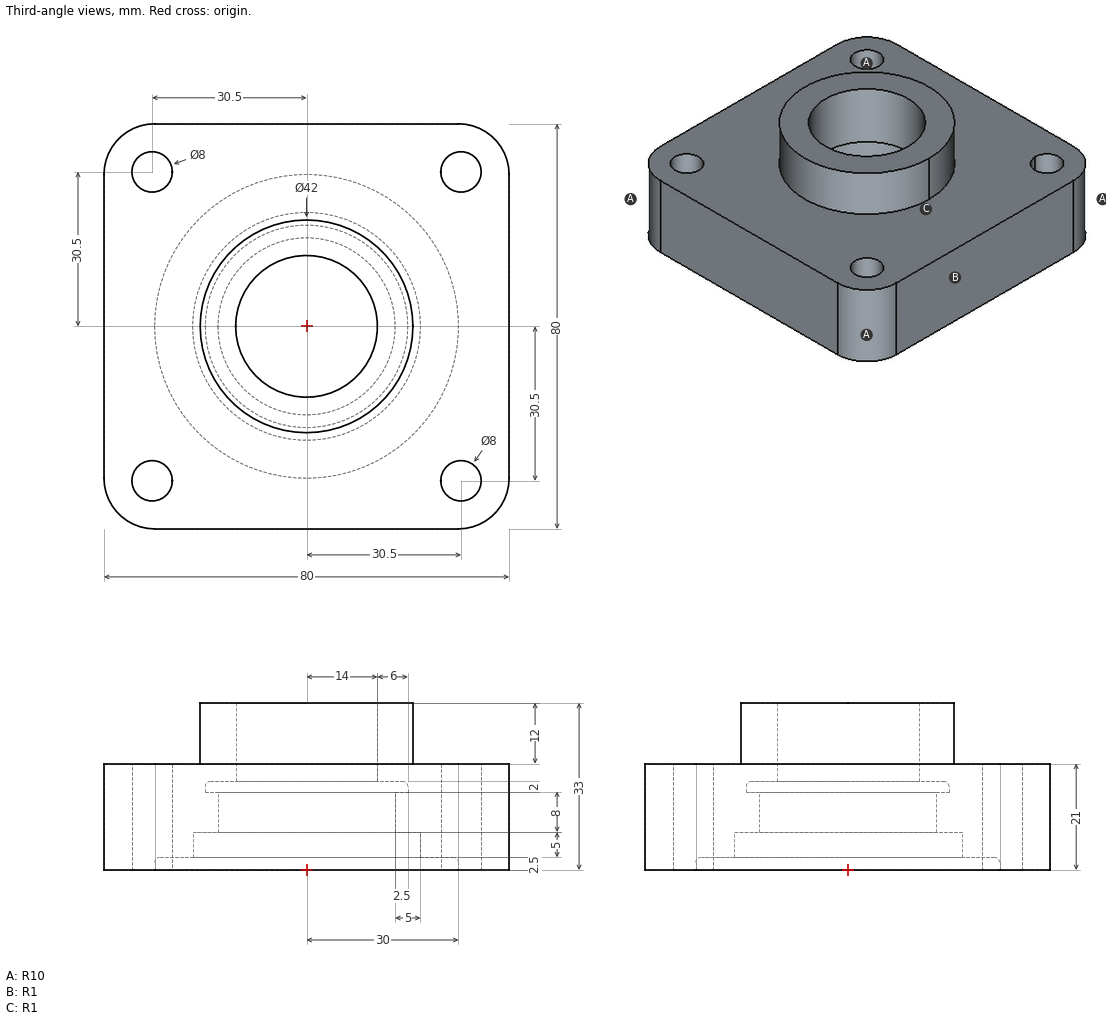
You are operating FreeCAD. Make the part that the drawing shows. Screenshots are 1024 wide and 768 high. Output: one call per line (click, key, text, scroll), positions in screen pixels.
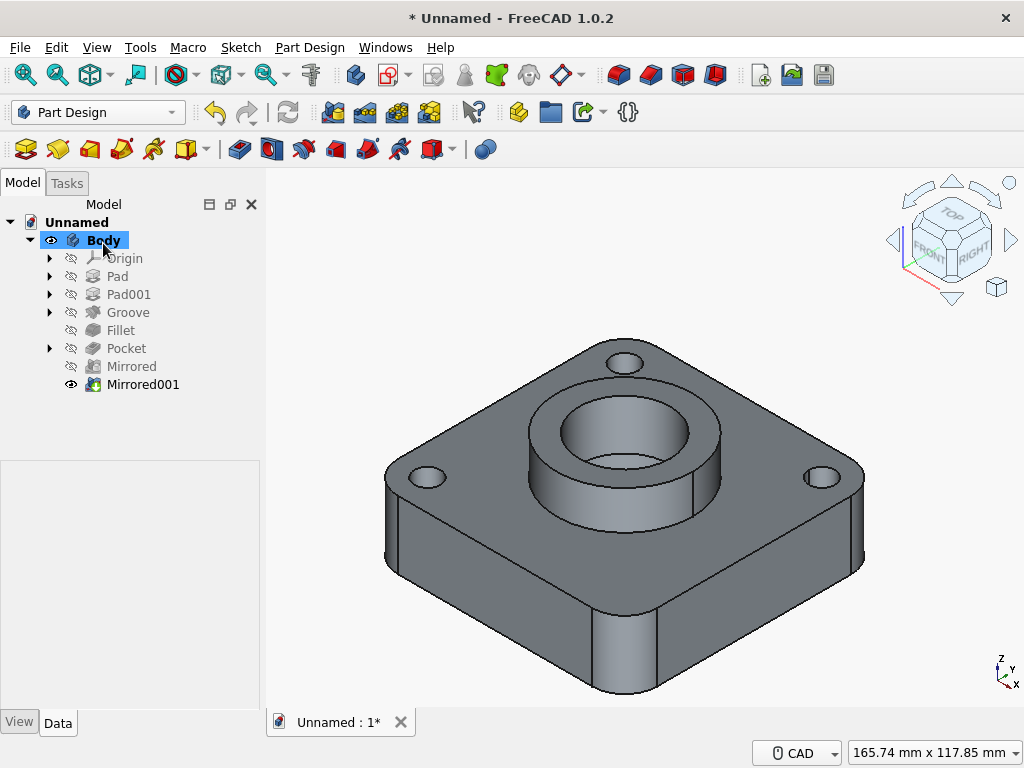
click(625, 562)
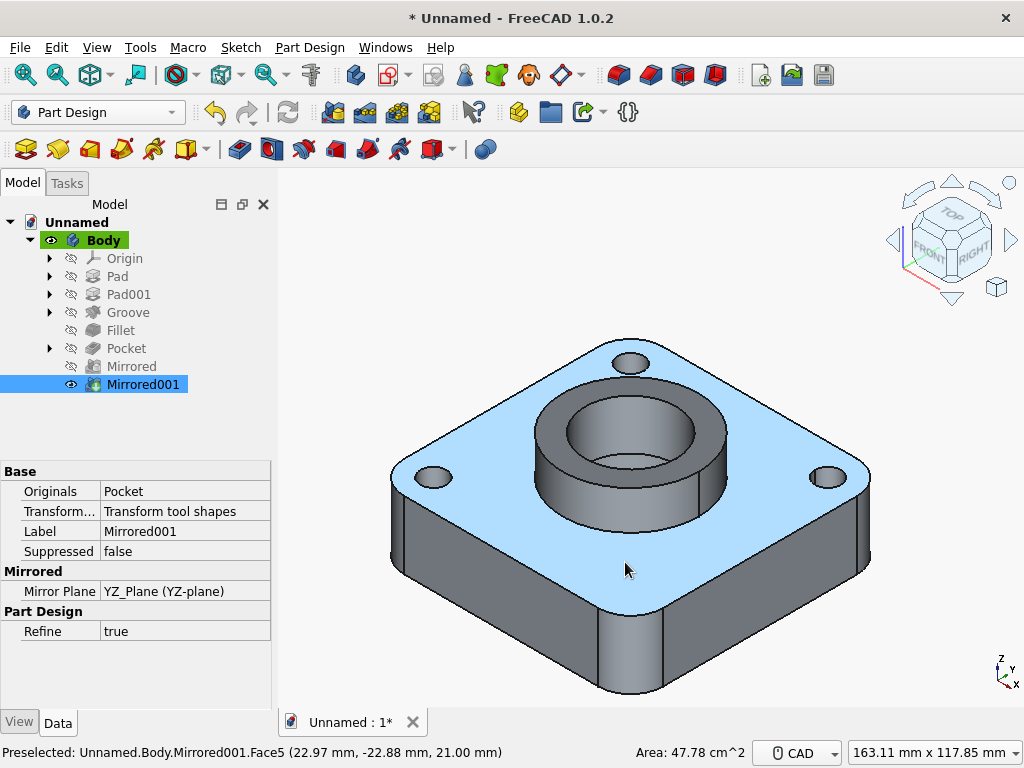
click(388, 76)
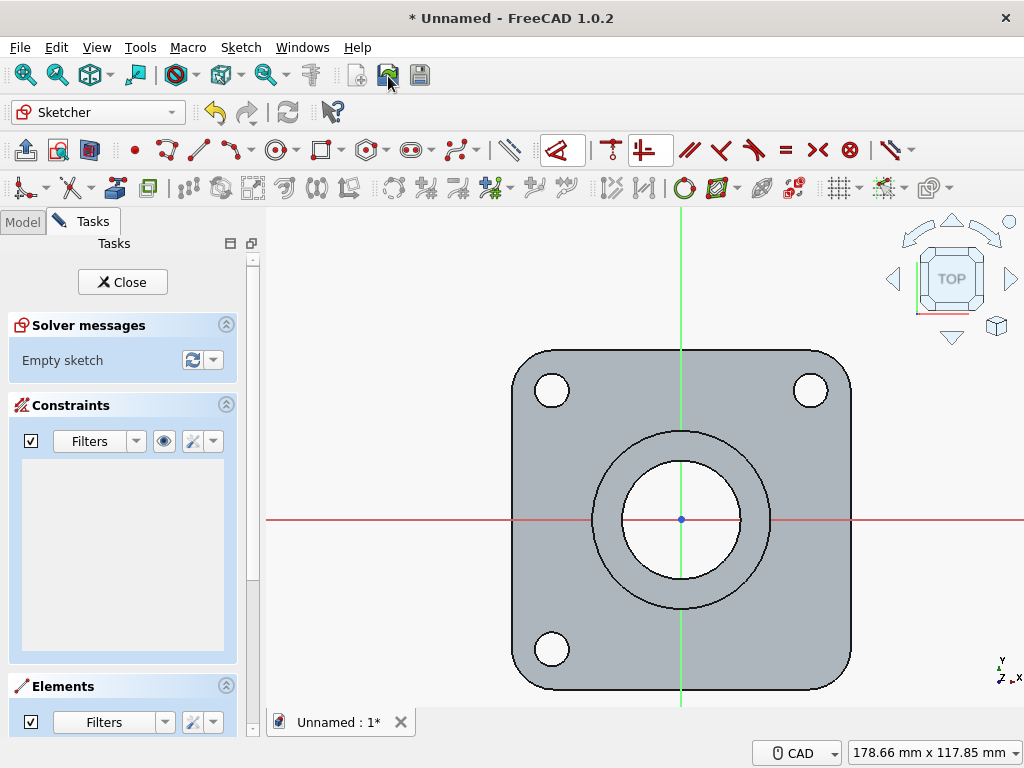
click(90, 150)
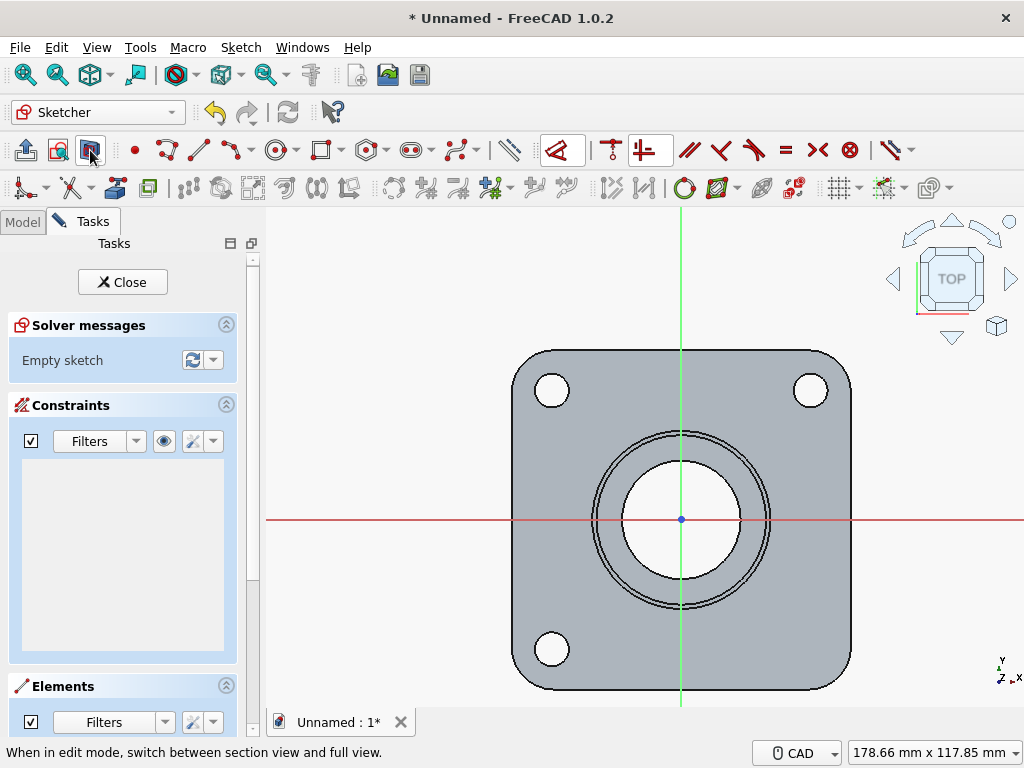
scroll(840, 673, up, 11)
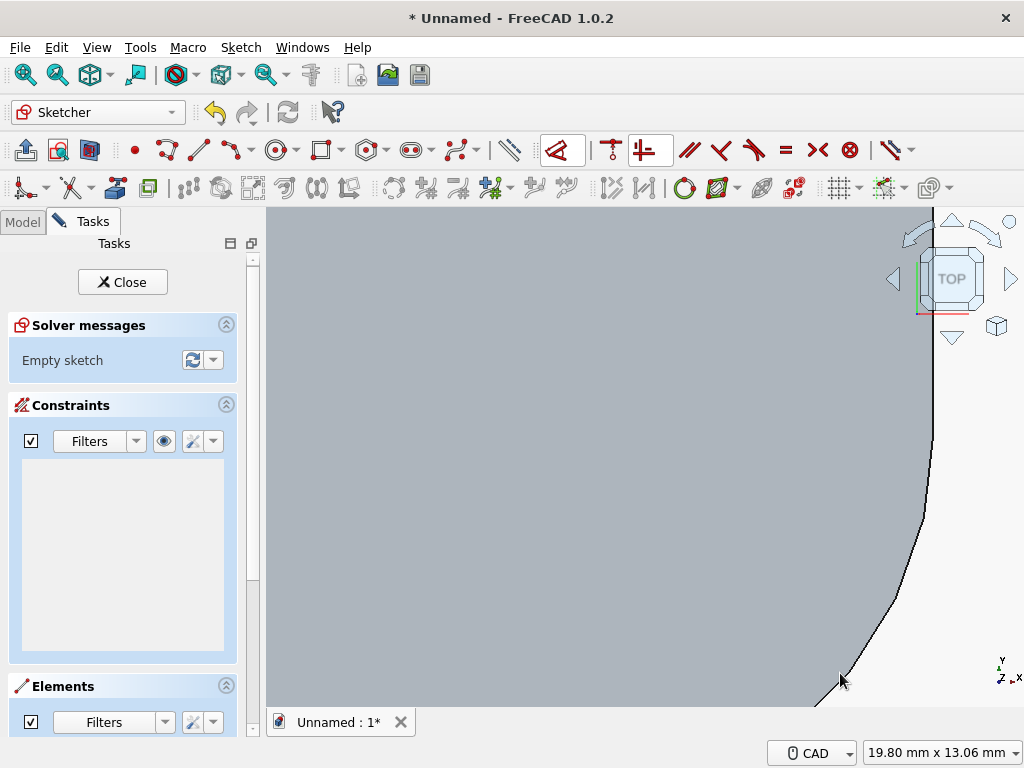
click(276, 150)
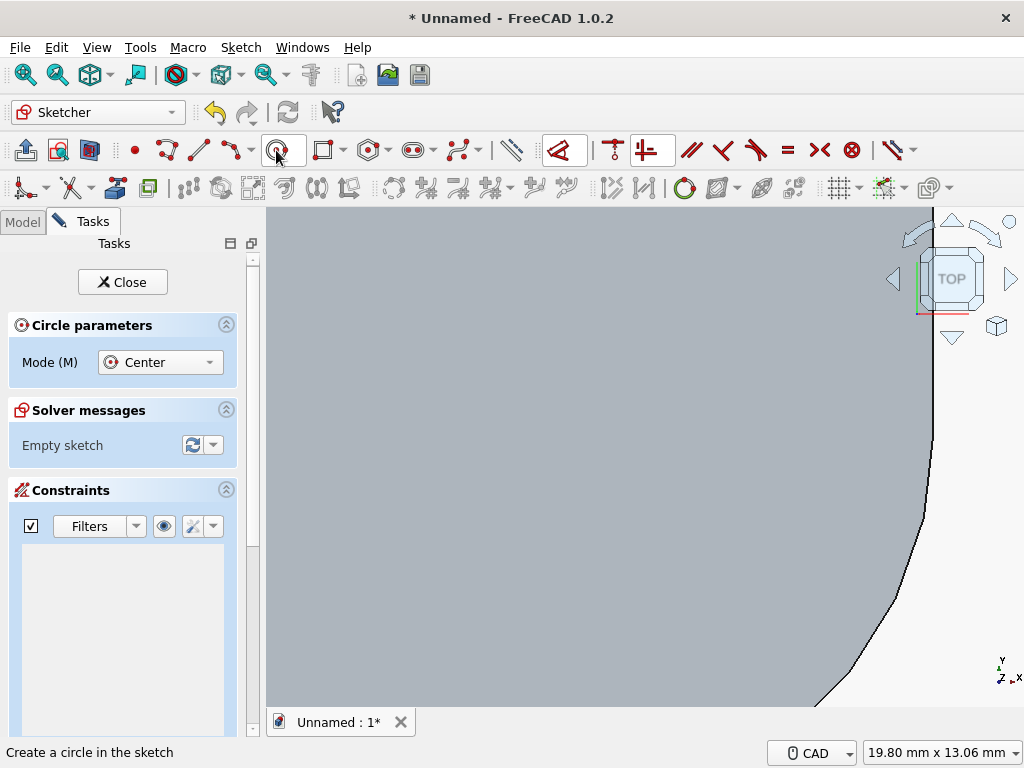
click(570, 452)
move(678, 343)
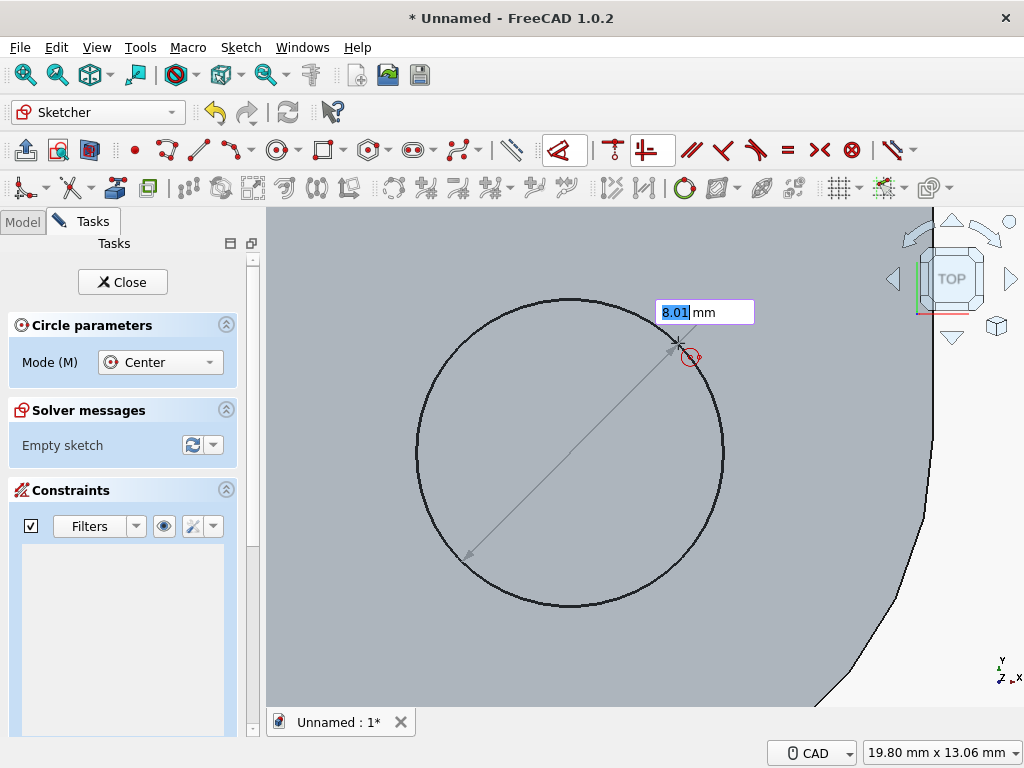
text(8)
key(Return)
key(Escape)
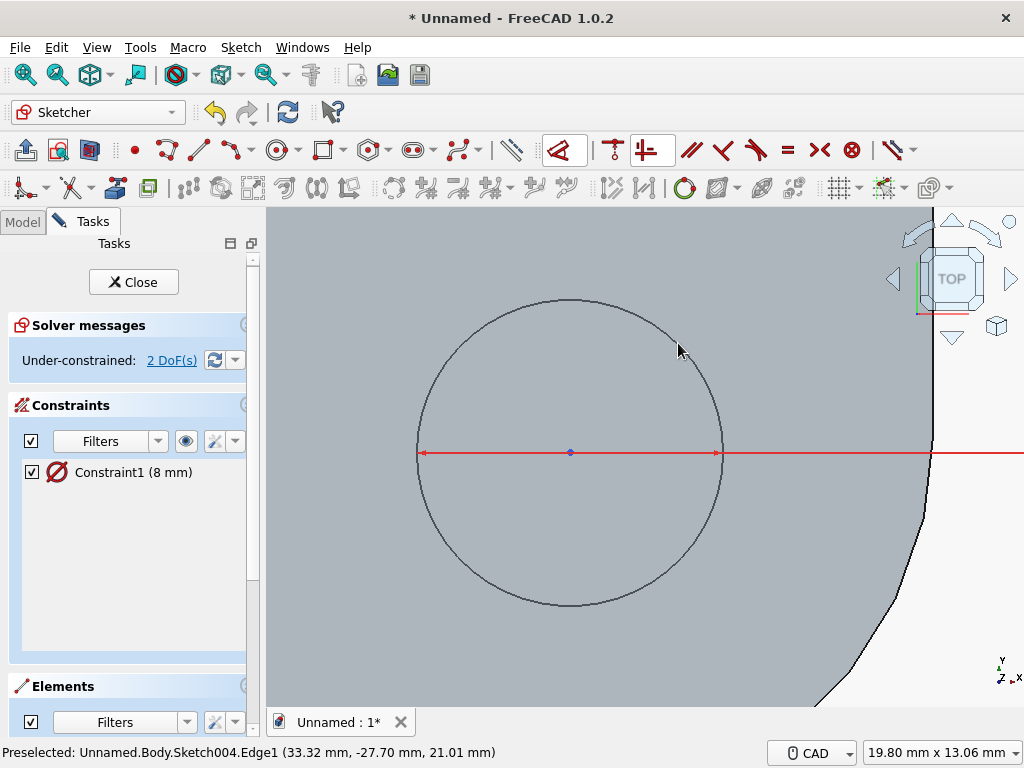
click(570, 453)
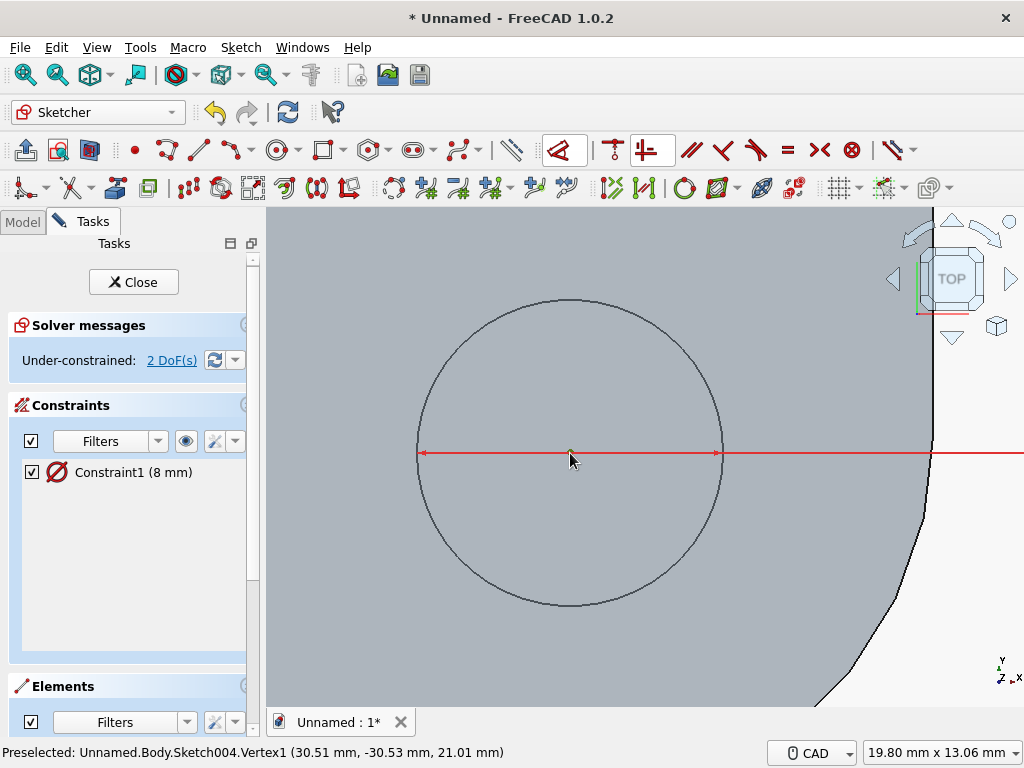
key(l)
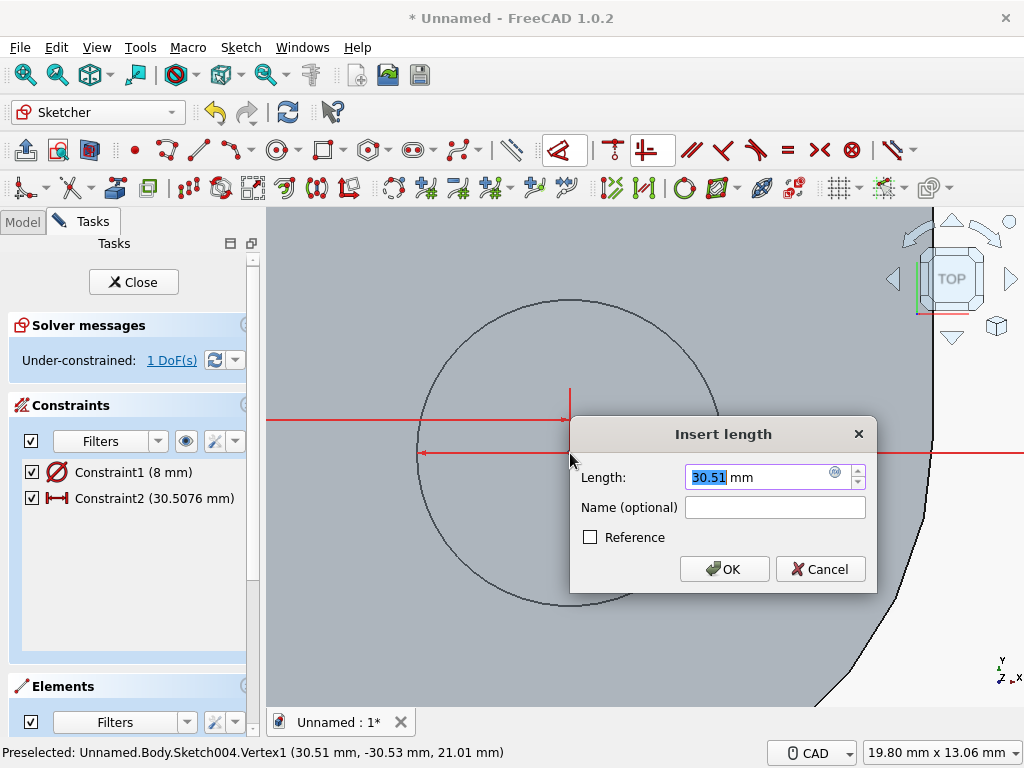
text(30.5)
key(Return)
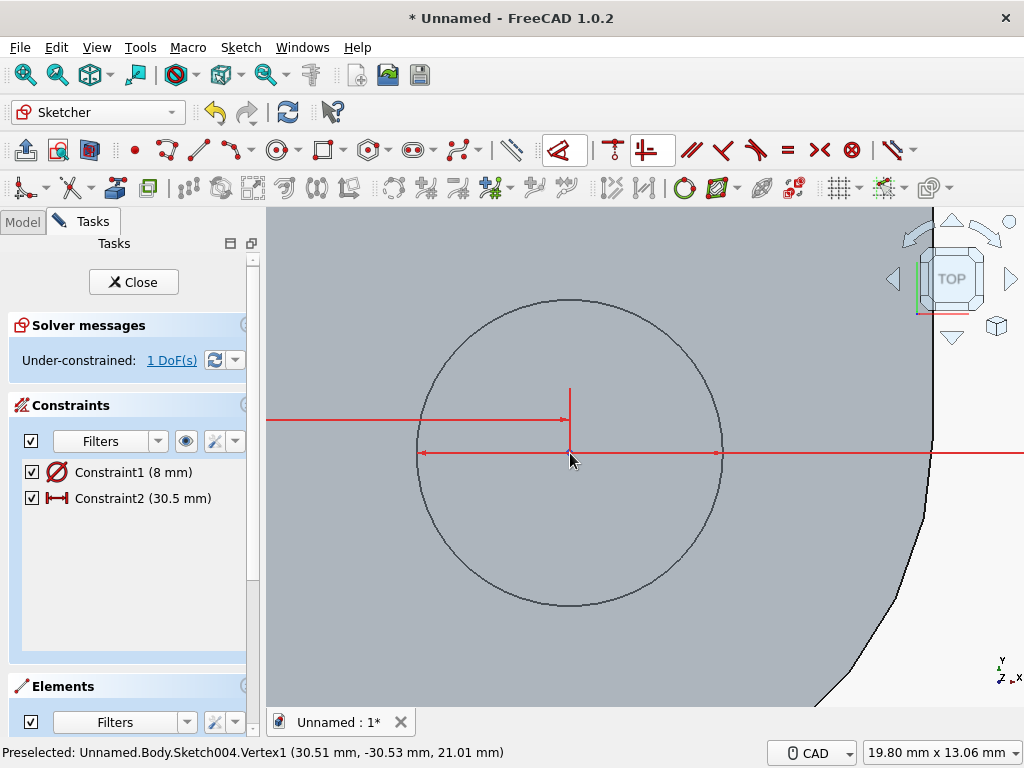
click(570, 453)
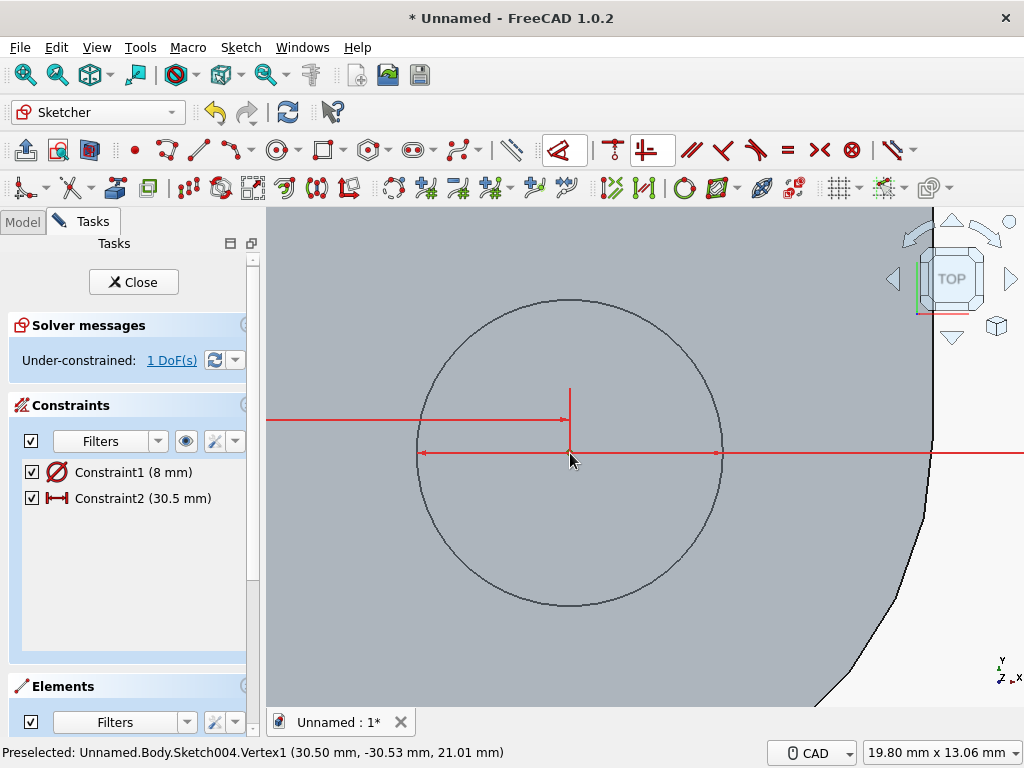
click(582, 150)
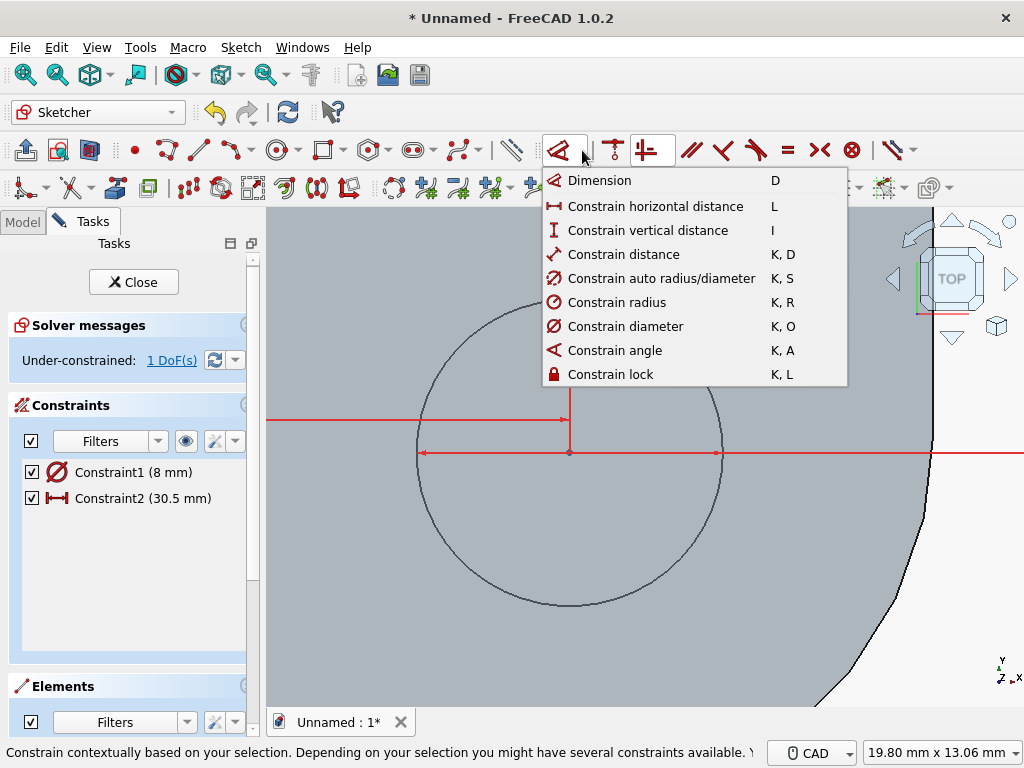
click(695, 230)